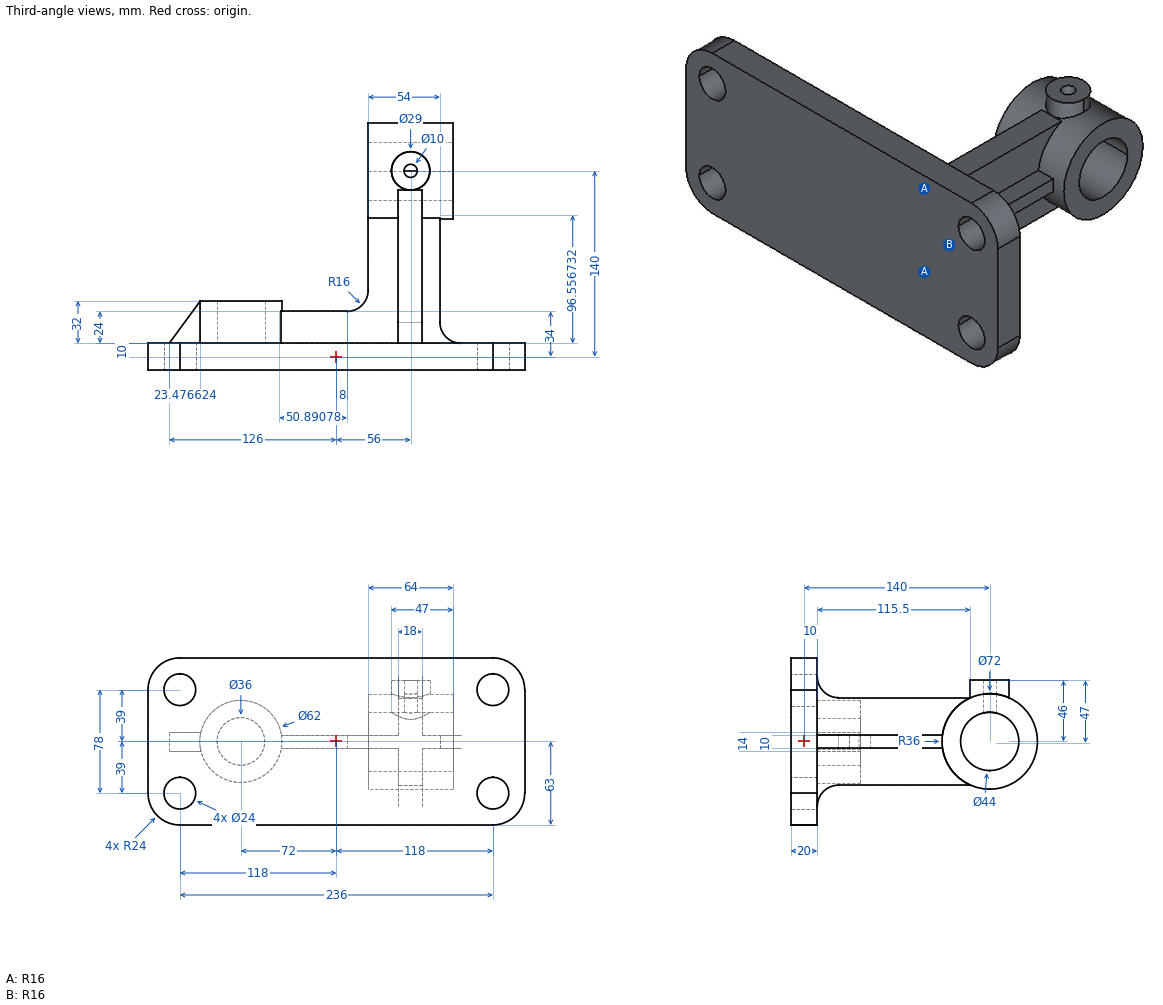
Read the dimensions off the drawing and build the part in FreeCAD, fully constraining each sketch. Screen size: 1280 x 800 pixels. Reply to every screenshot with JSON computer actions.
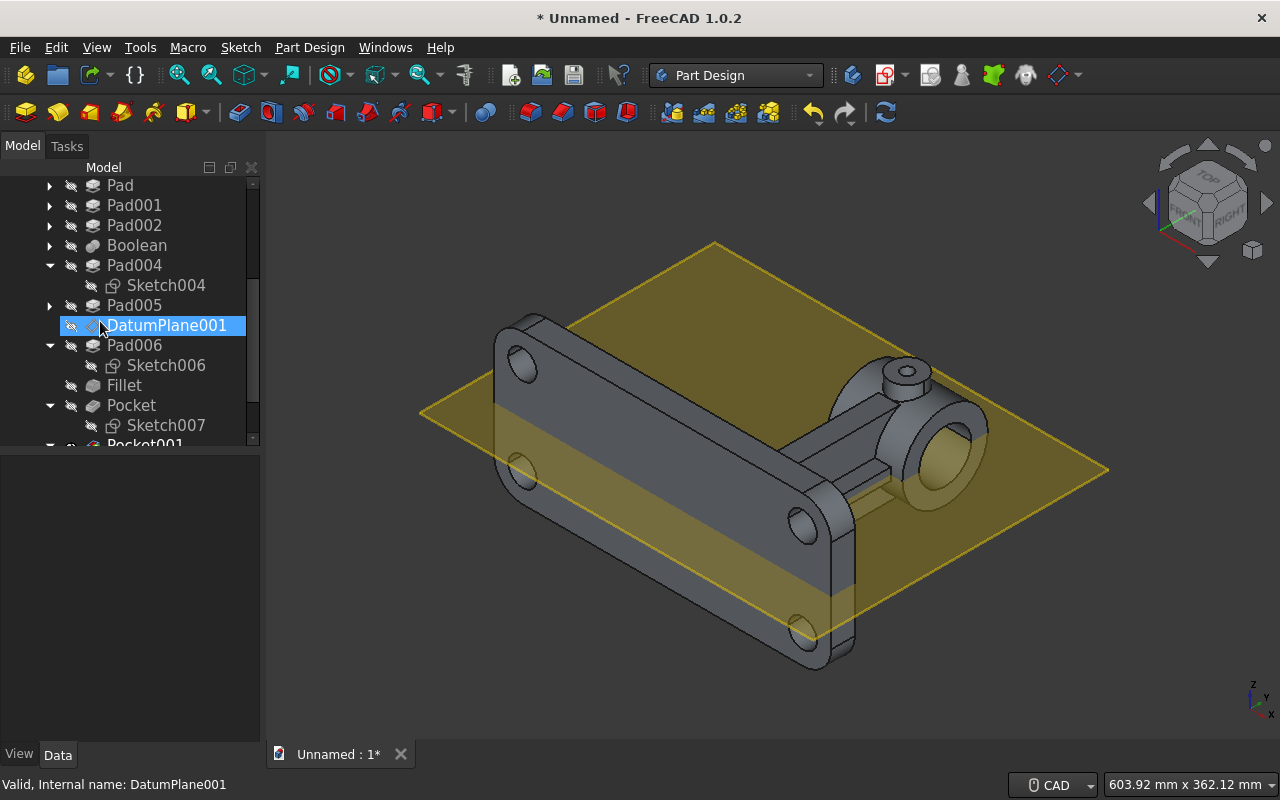
{"action": "scroll", "coordinate": [140, 321], "scroll_direction": "up", "scroll_amount": 15}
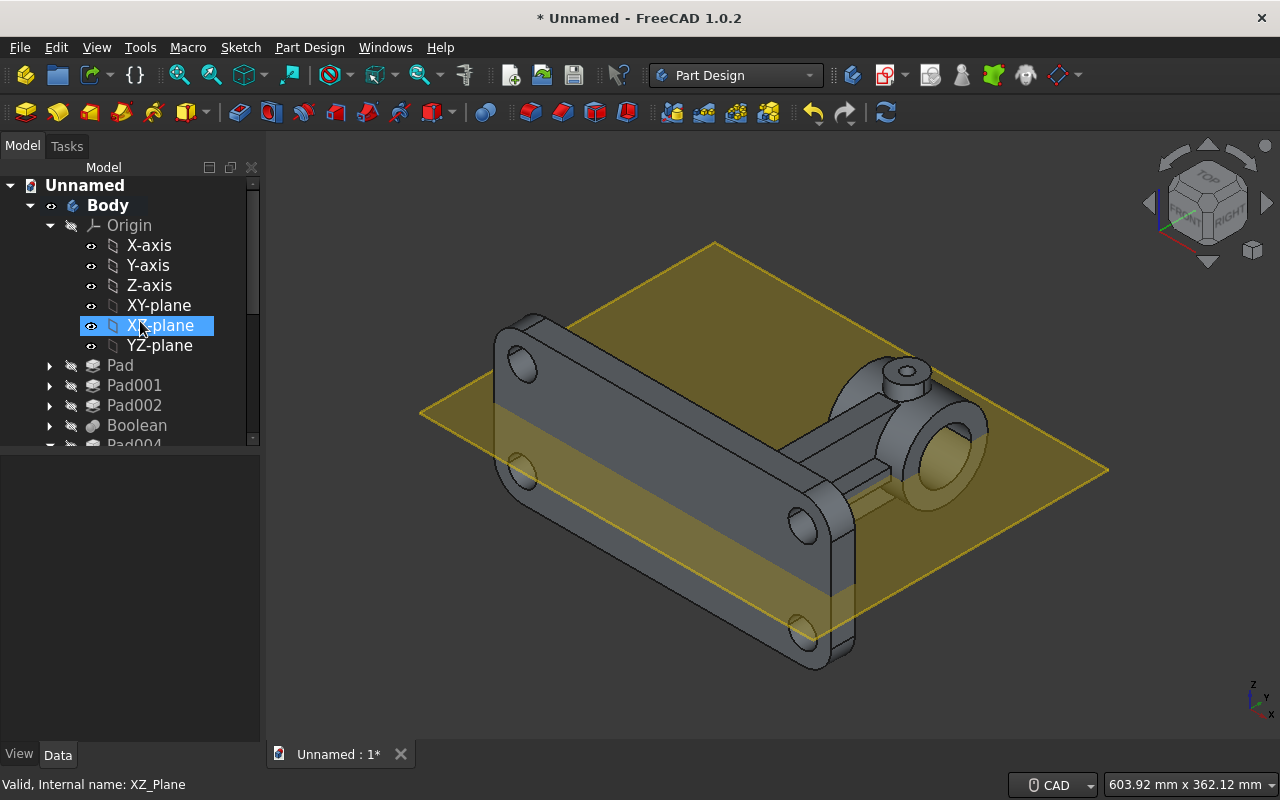
{"action": "scroll", "coordinate": [100, 321], "scroll_direction": "down", "scroll_amount": 6}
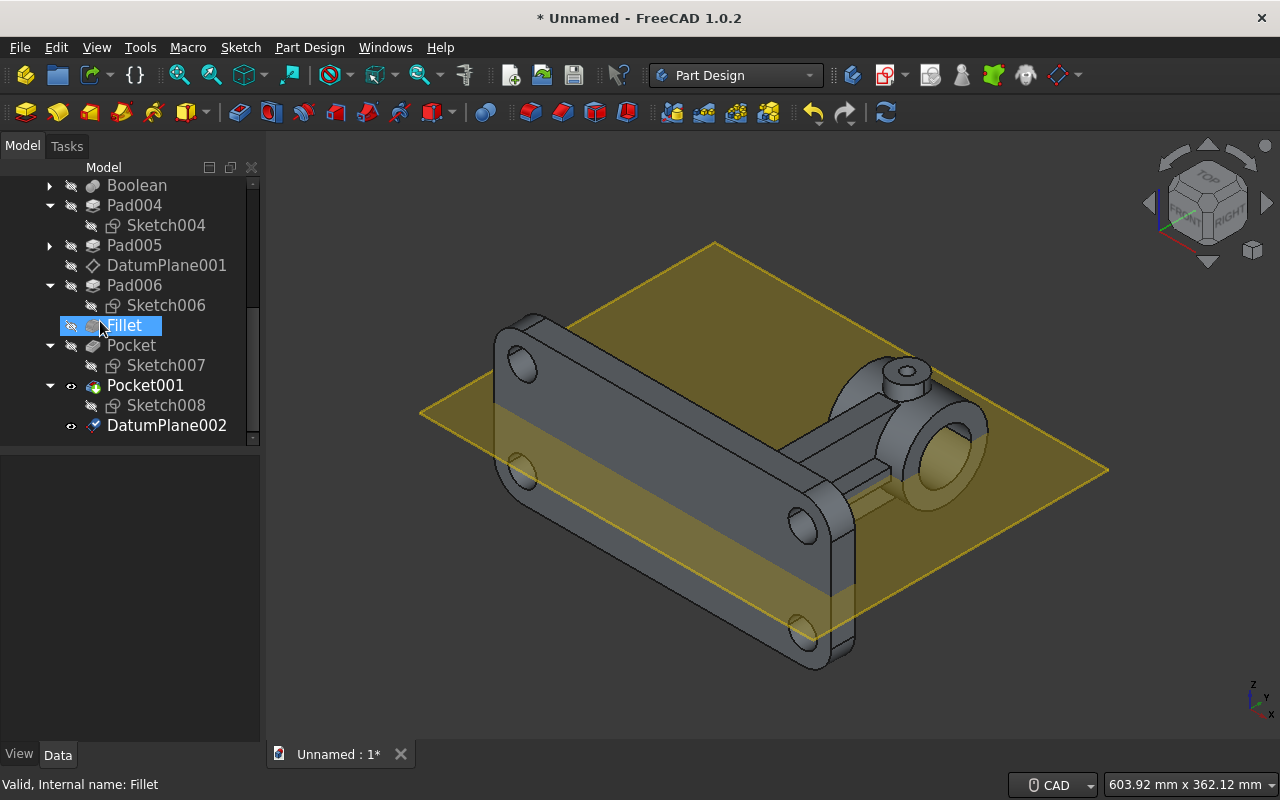
{"action": "left_click", "coordinate": [116, 426]}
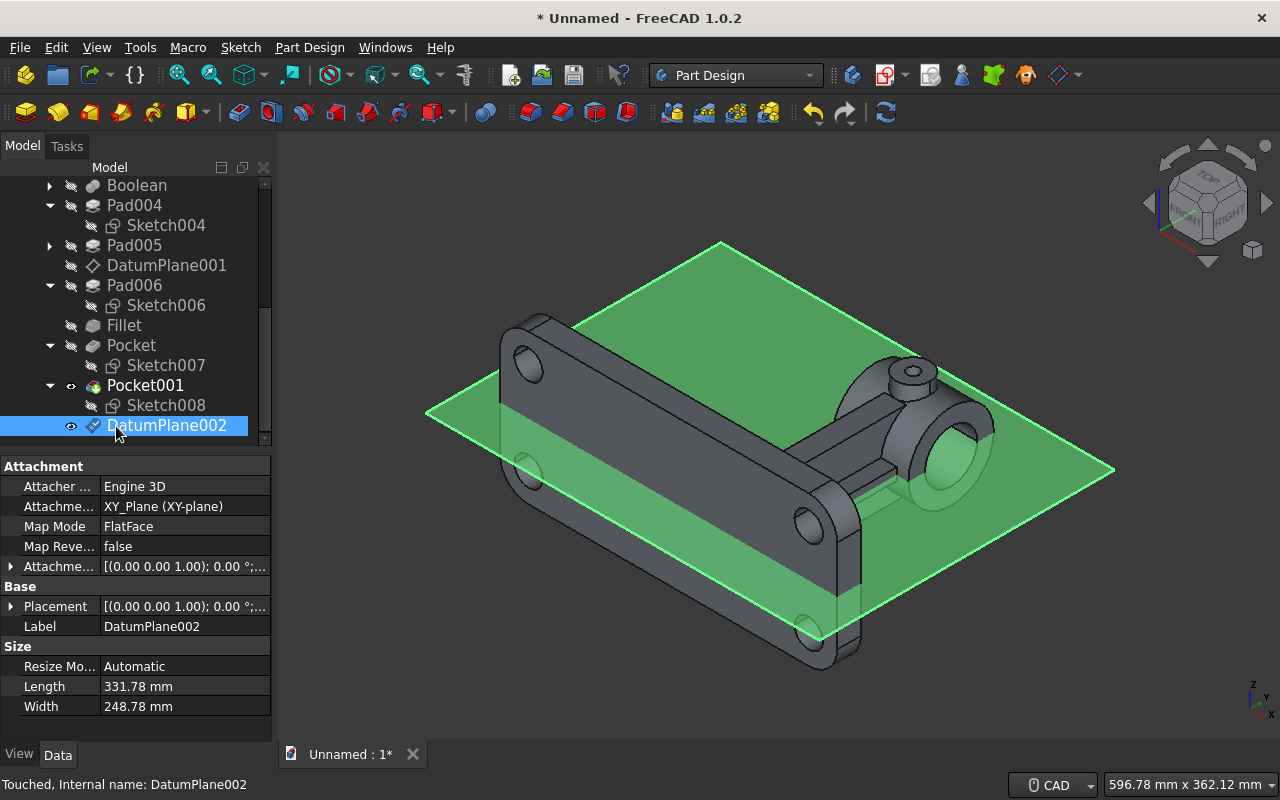
{"action": "left_click", "coordinate": [886, 76]}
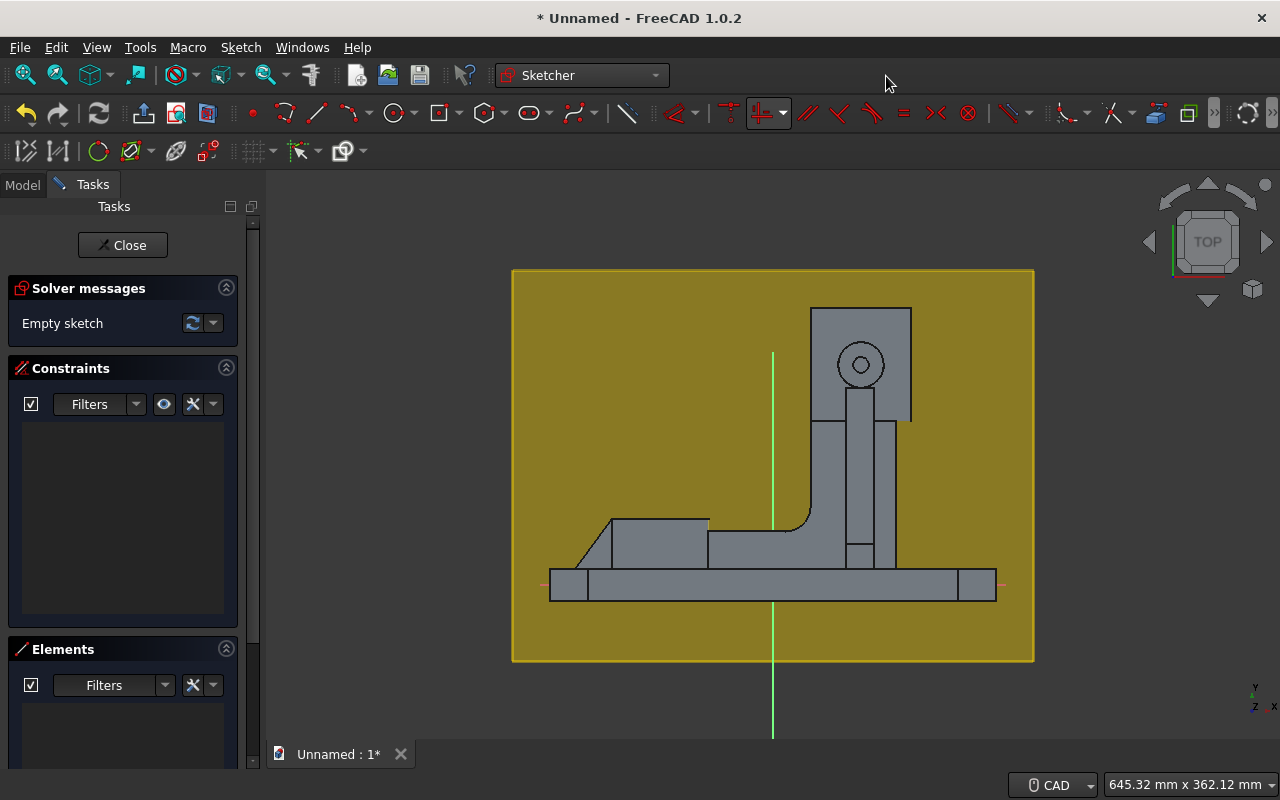
{"action": "left_click", "coordinate": [208, 114]}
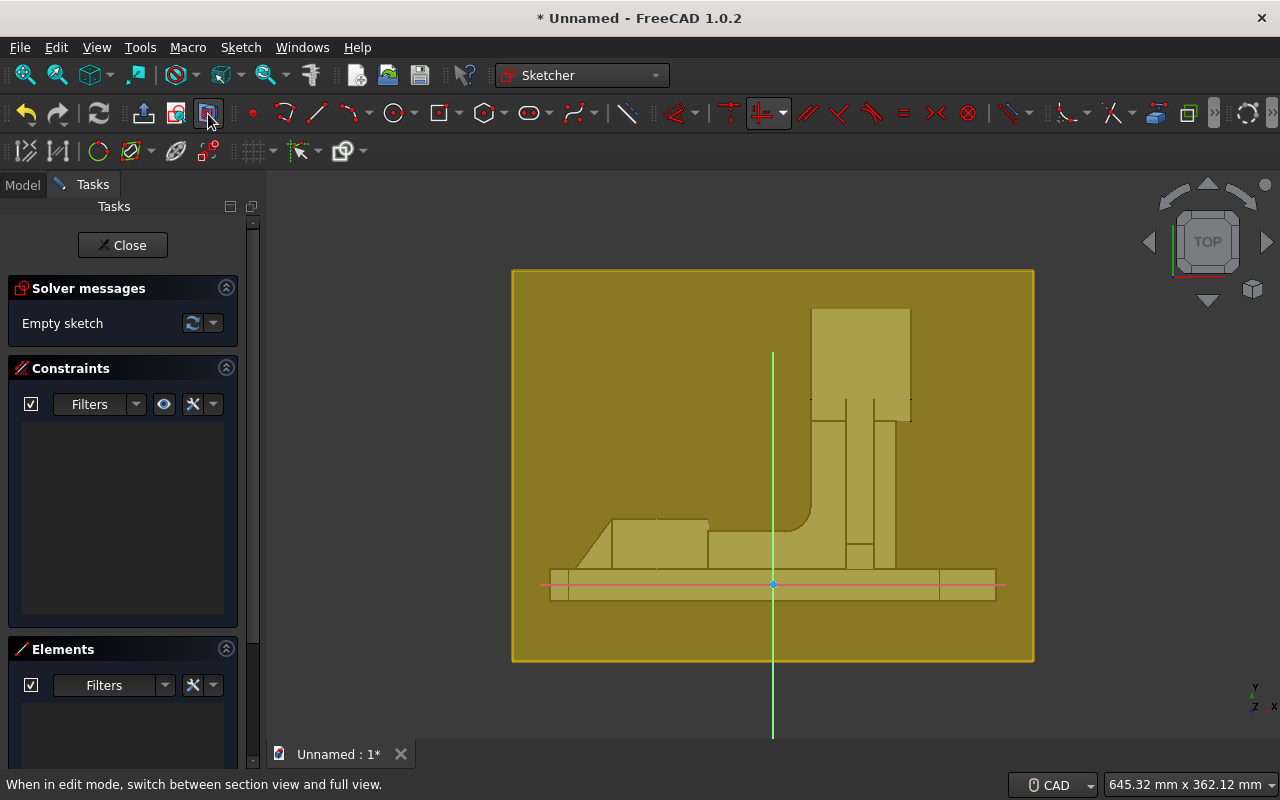
{"action": "scroll", "coordinate": [869, 360], "scroll_direction": "up", "scroll_amount": 15}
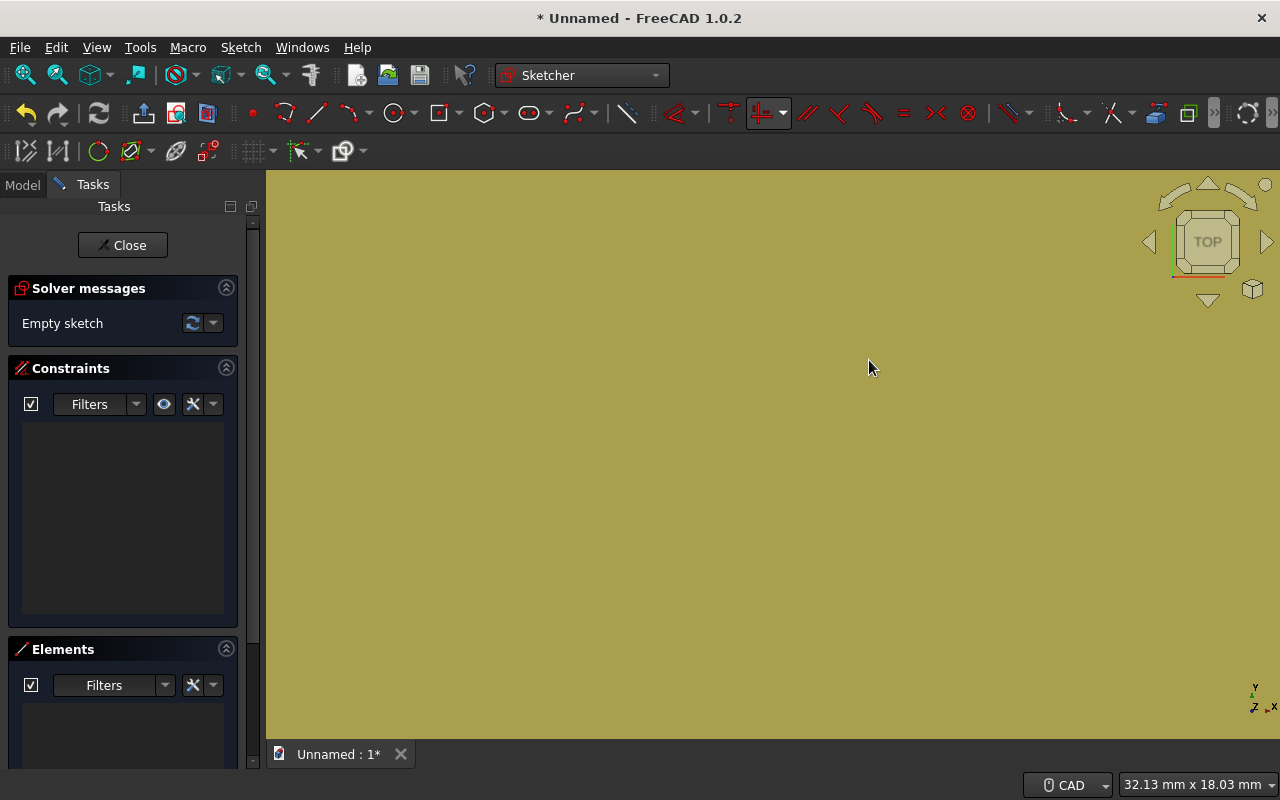
{"action": "left_click", "coordinate": [394, 114]}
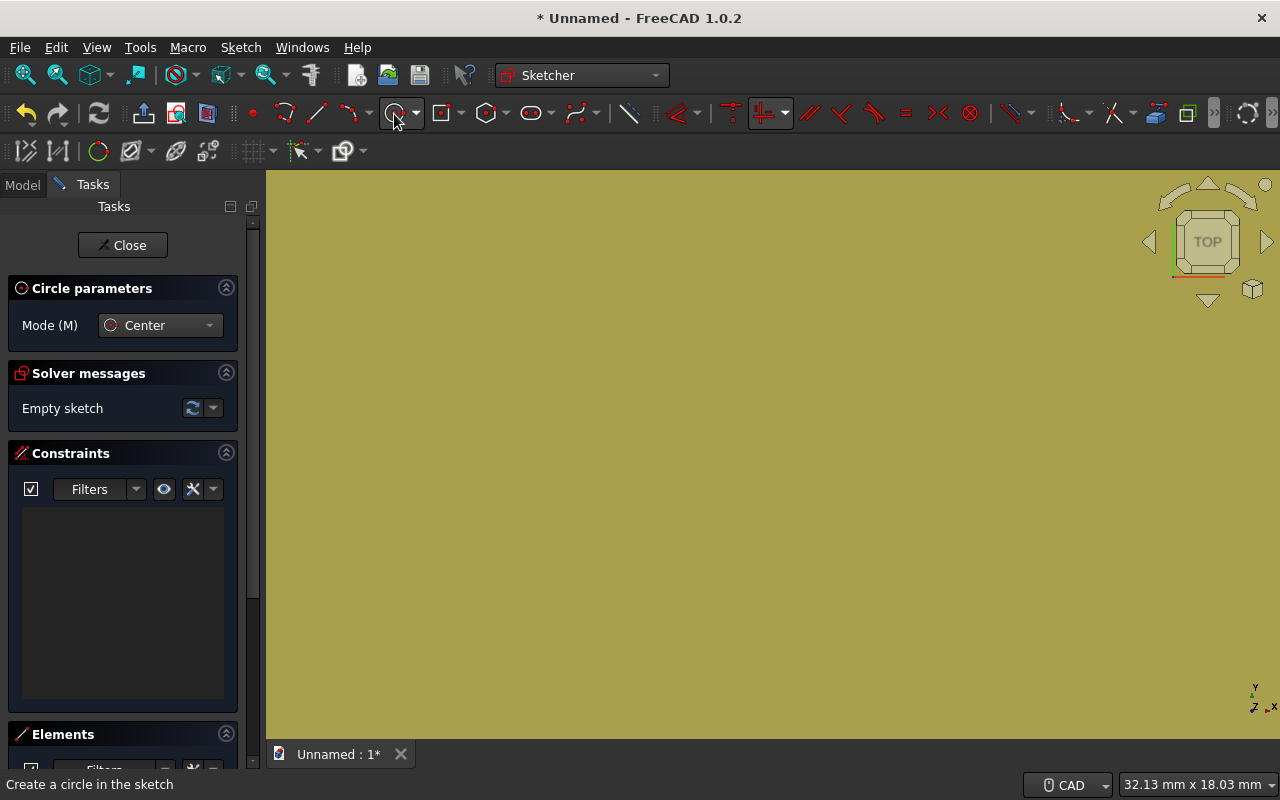
{"action": "left_click", "coordinate": [697, 453]}
{"action": "mouse_move", "coordinate": [808, 341]}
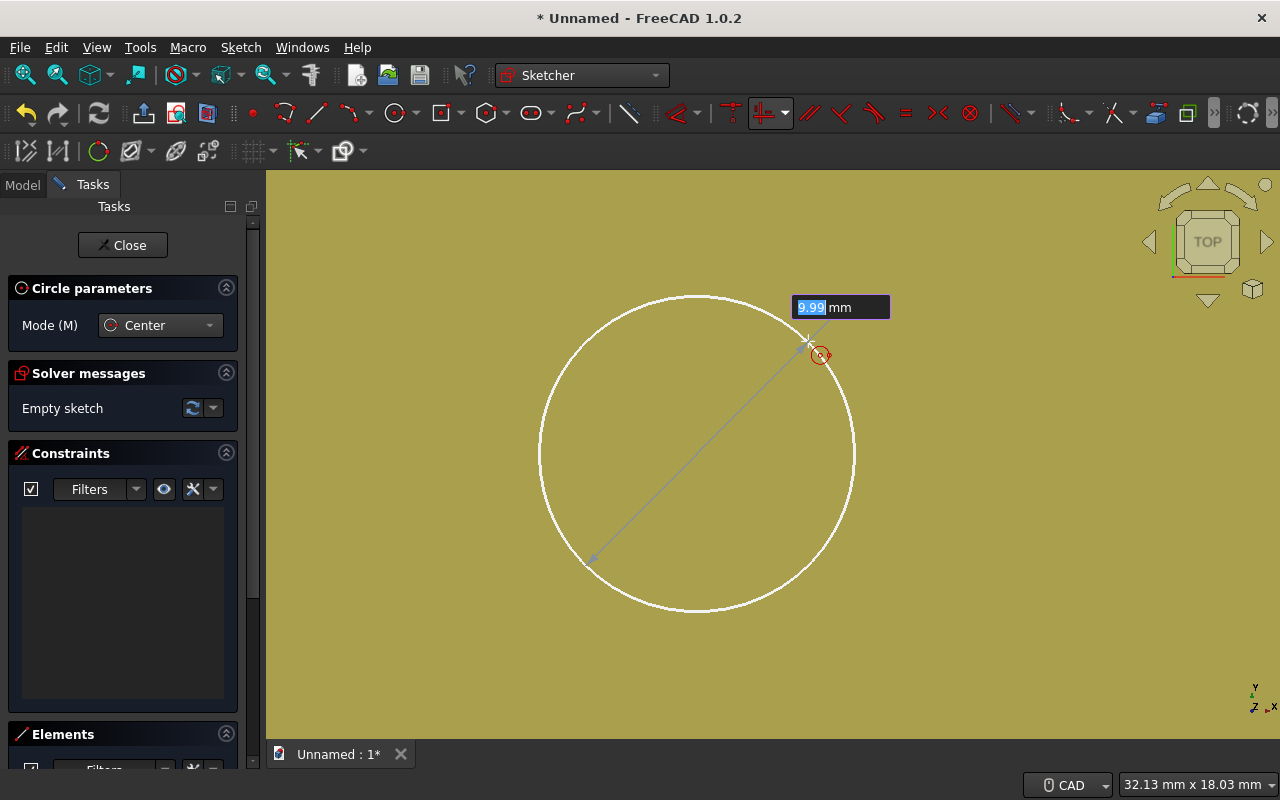
{"action": "type", "text": "10"}
{"action": "key", "text": "Return"}
{"action": "key", "text": "Escape"}